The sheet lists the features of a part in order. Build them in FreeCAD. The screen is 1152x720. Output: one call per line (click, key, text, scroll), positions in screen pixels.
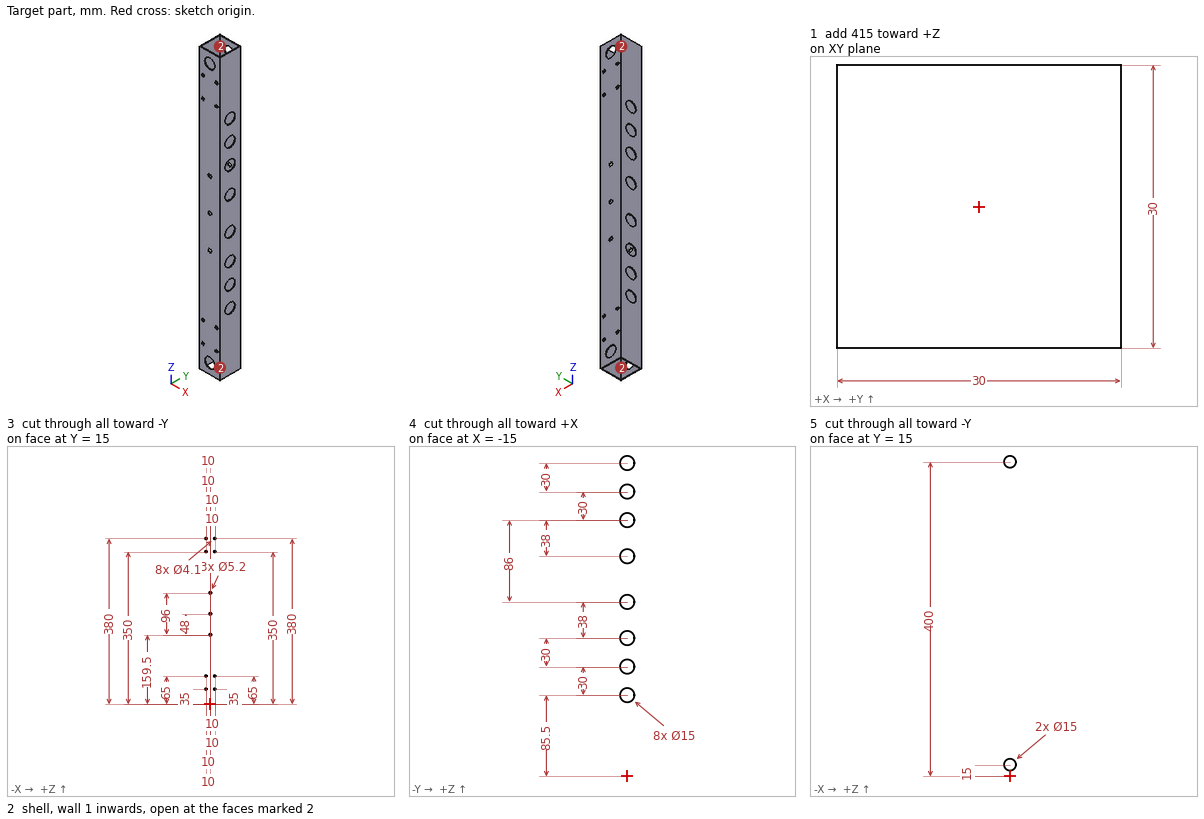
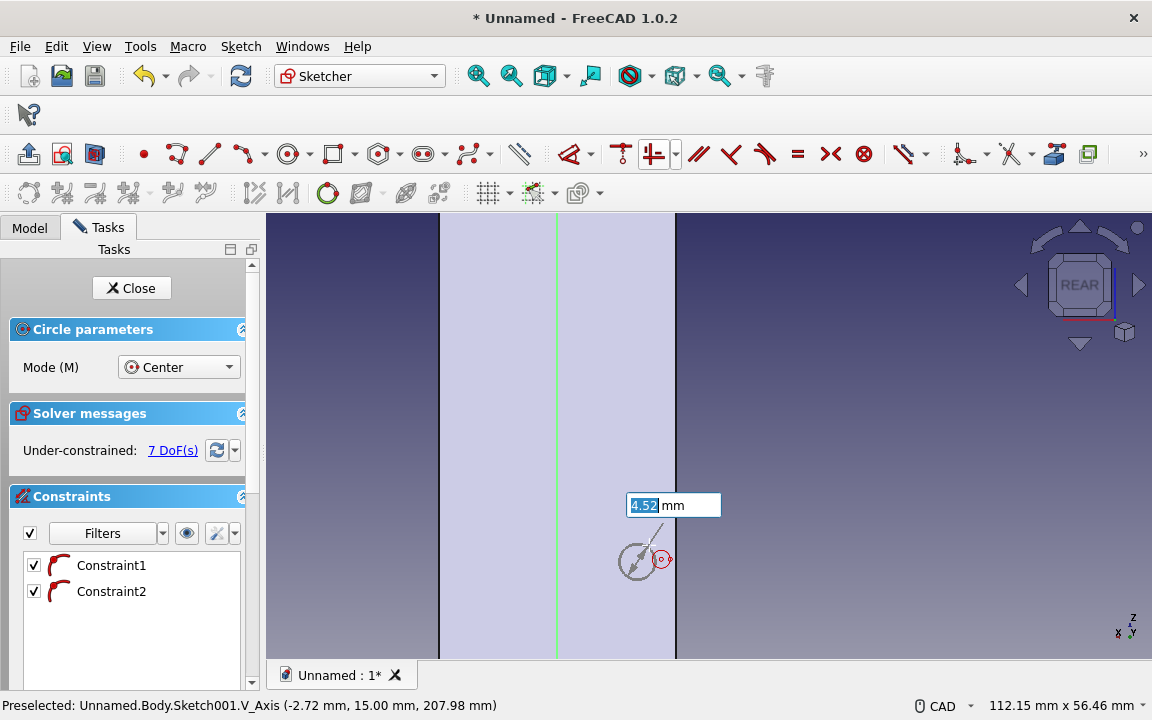
click(648, 544)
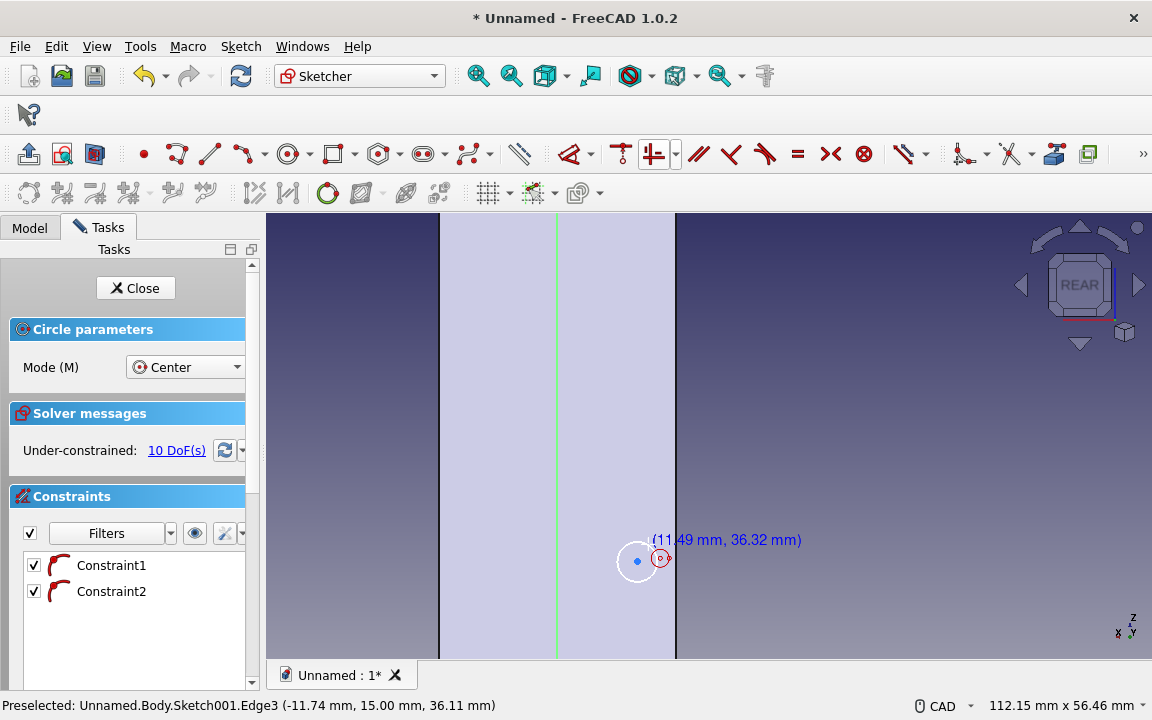
scroll(649, 547, down, 12)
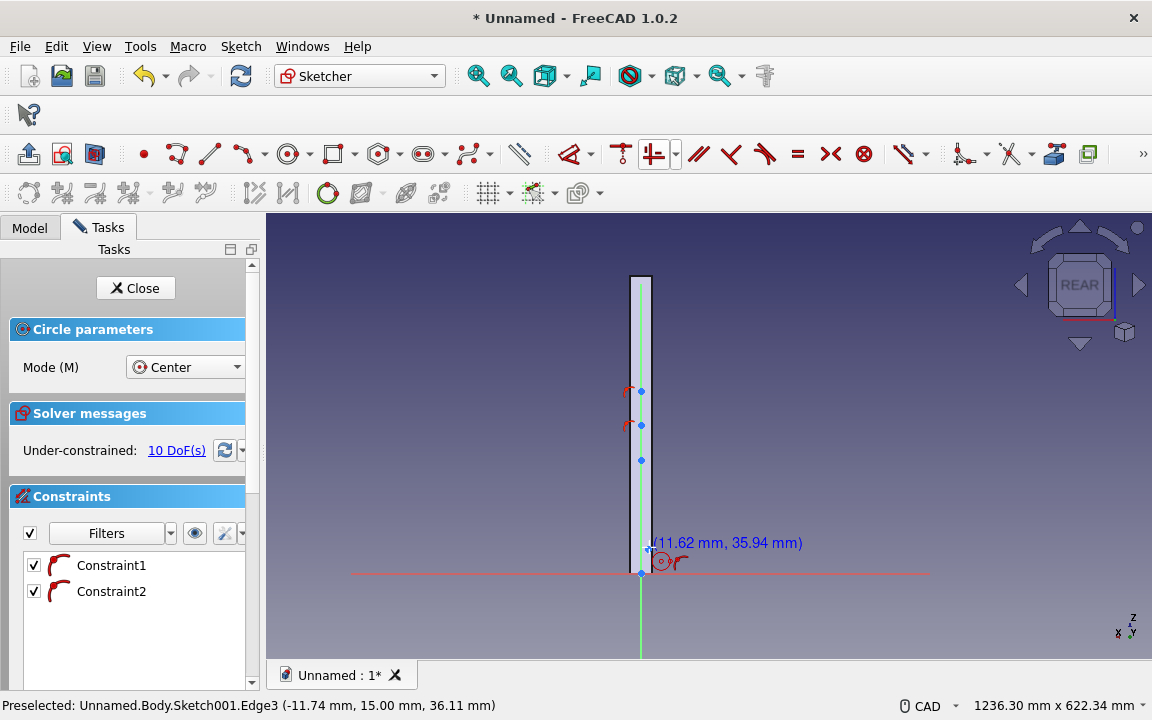
scroll(648, 301, up, 14)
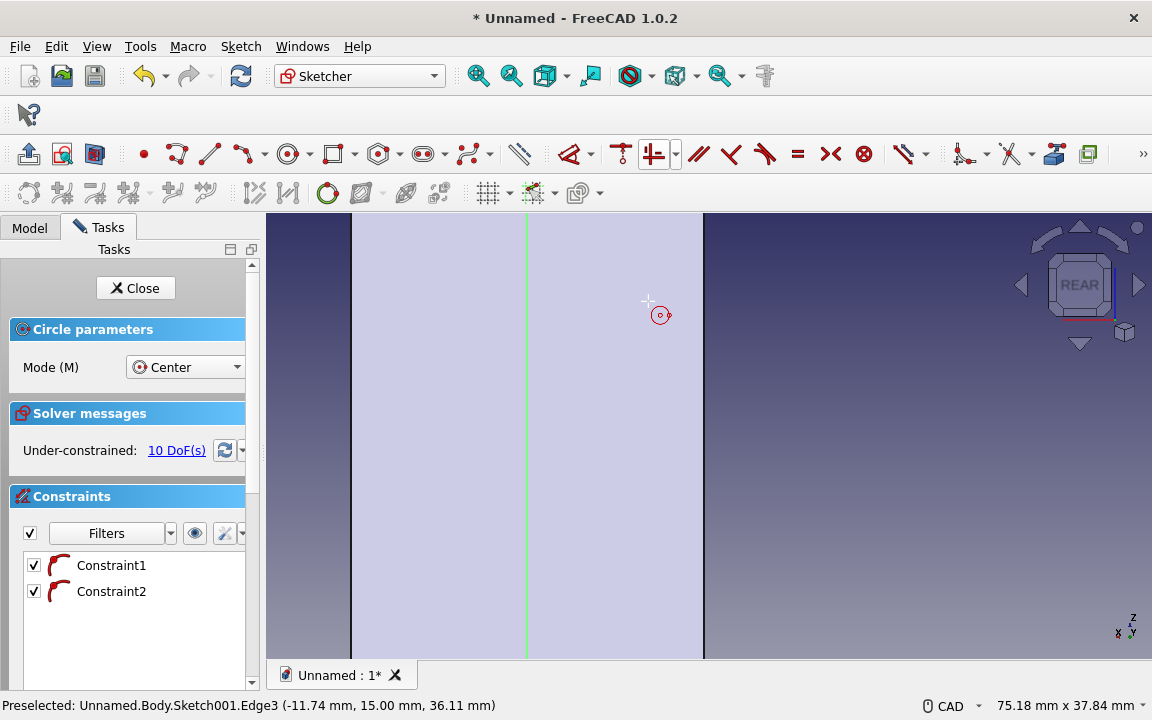
scroll(648, 301, down, 14)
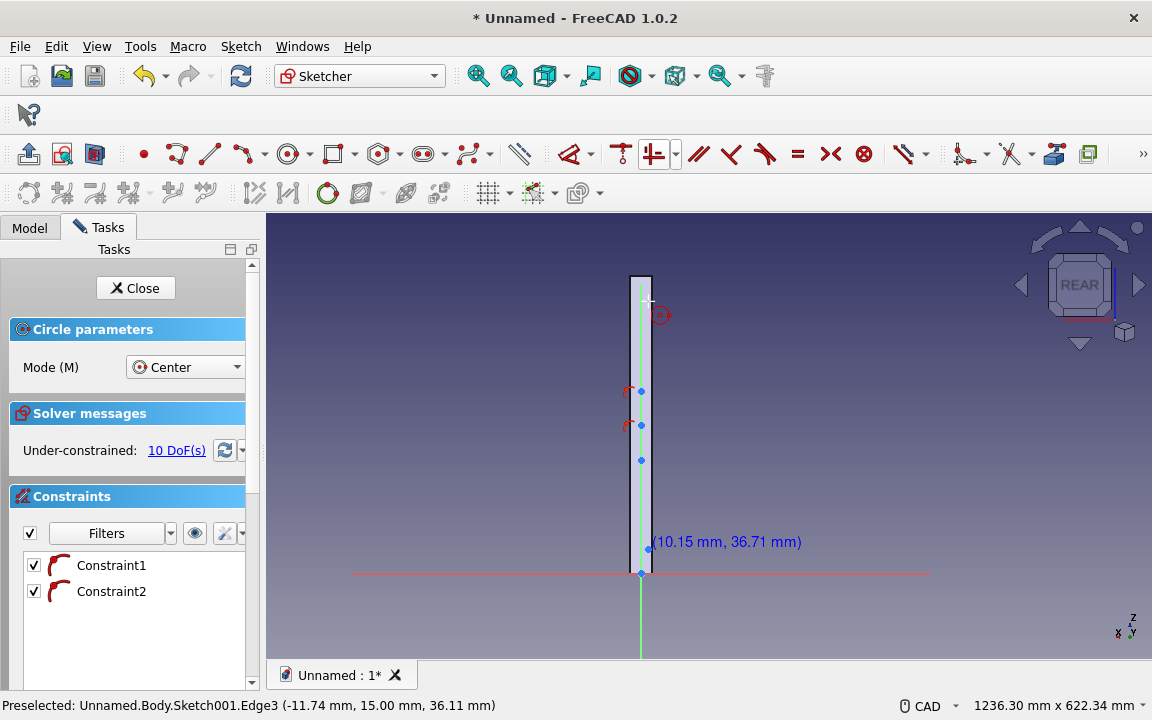
scroll(648, 301, up, 4)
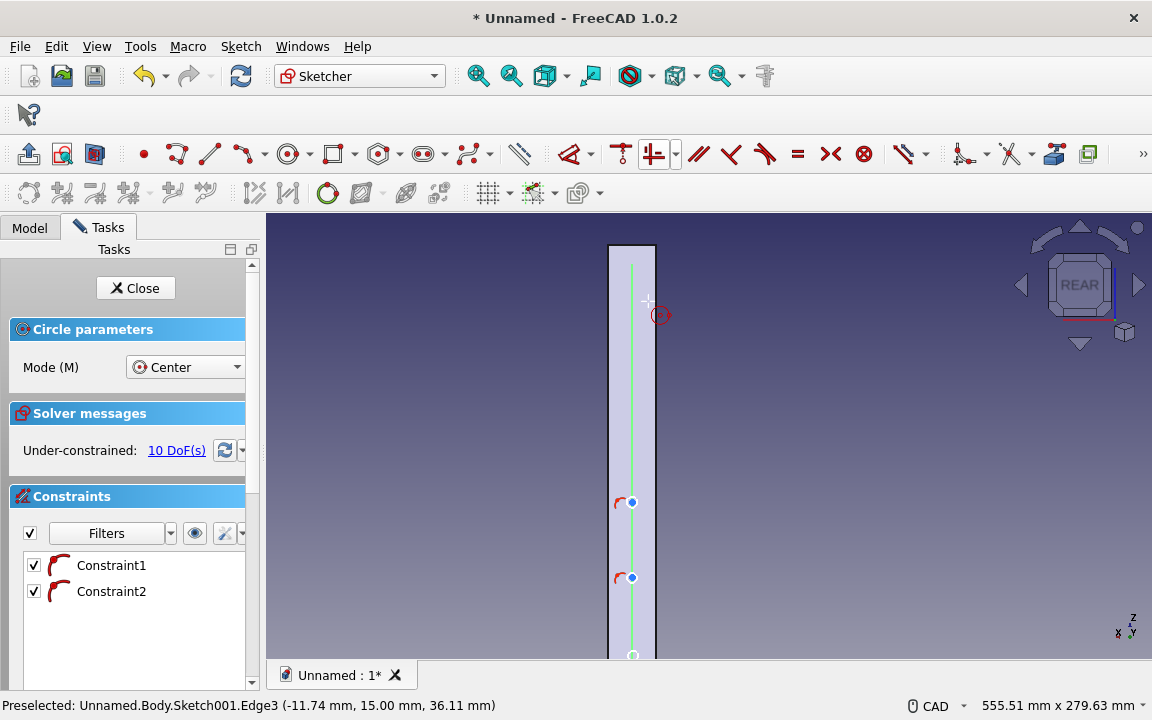
click(648, 301)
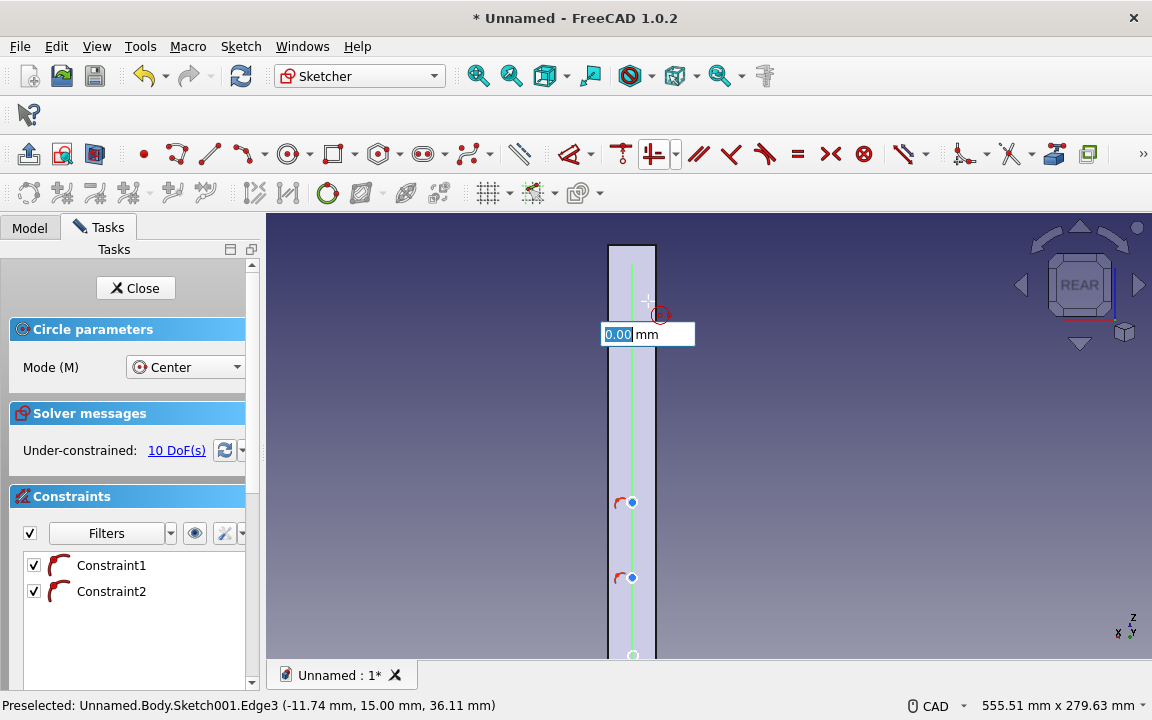
scroll(650, 299, up, 8)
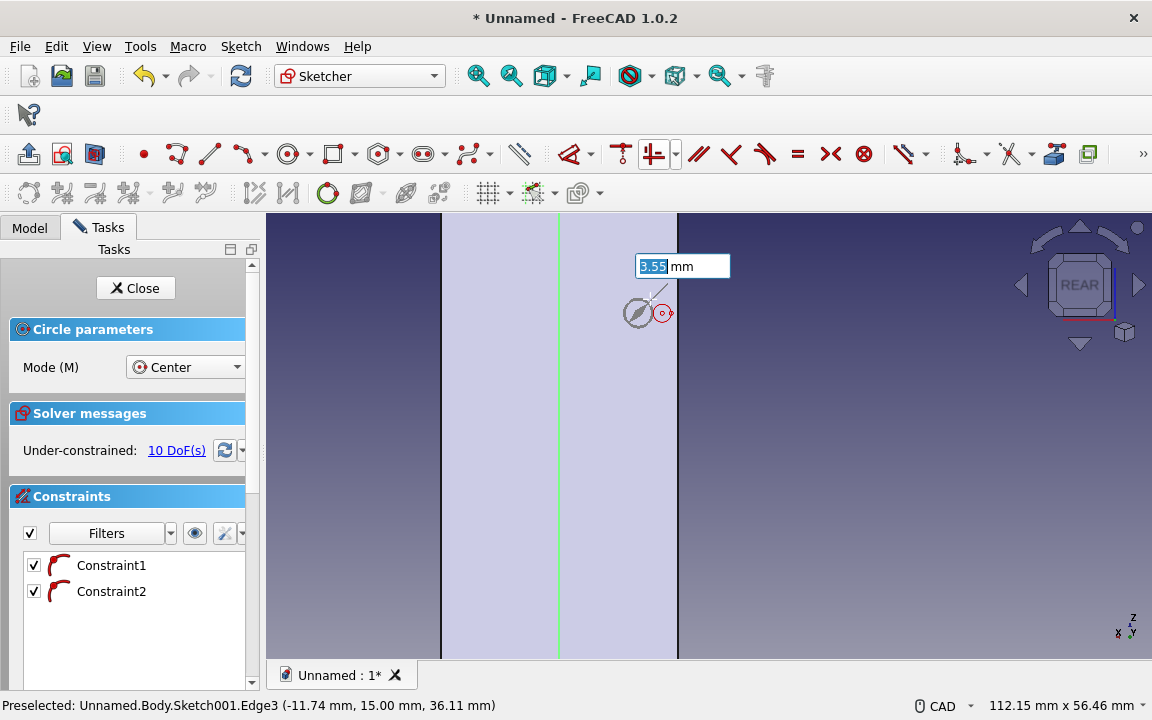
click(650, 298)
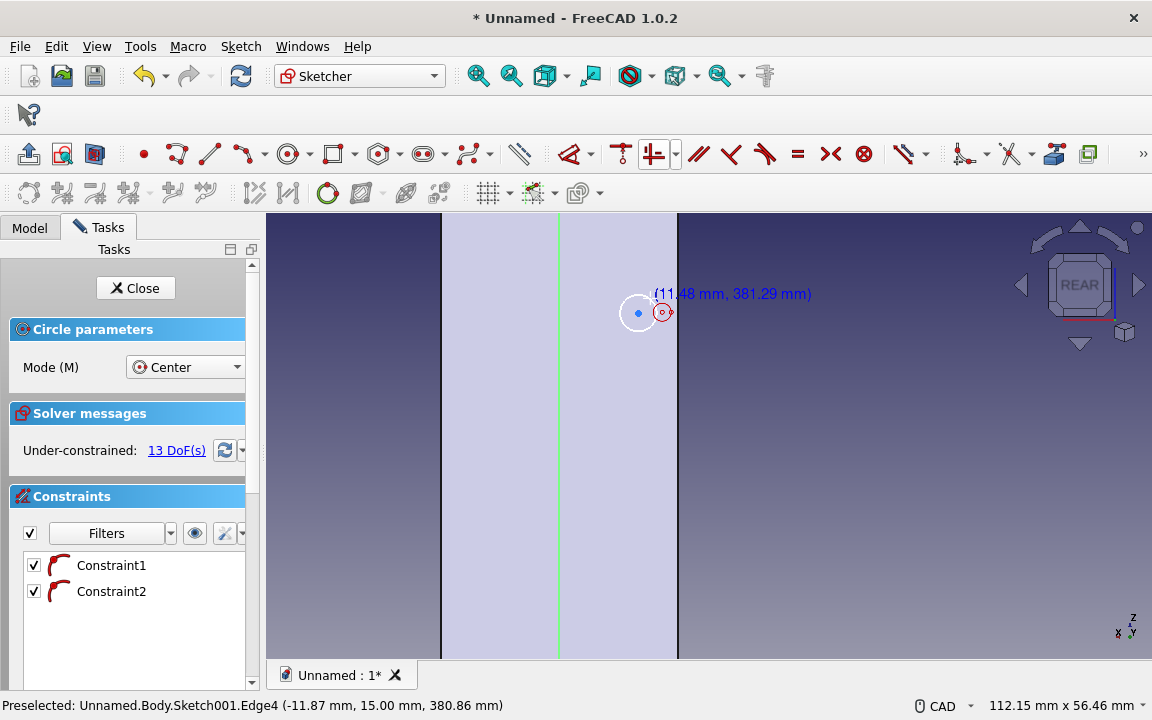
scroll(649, 300, down, 12)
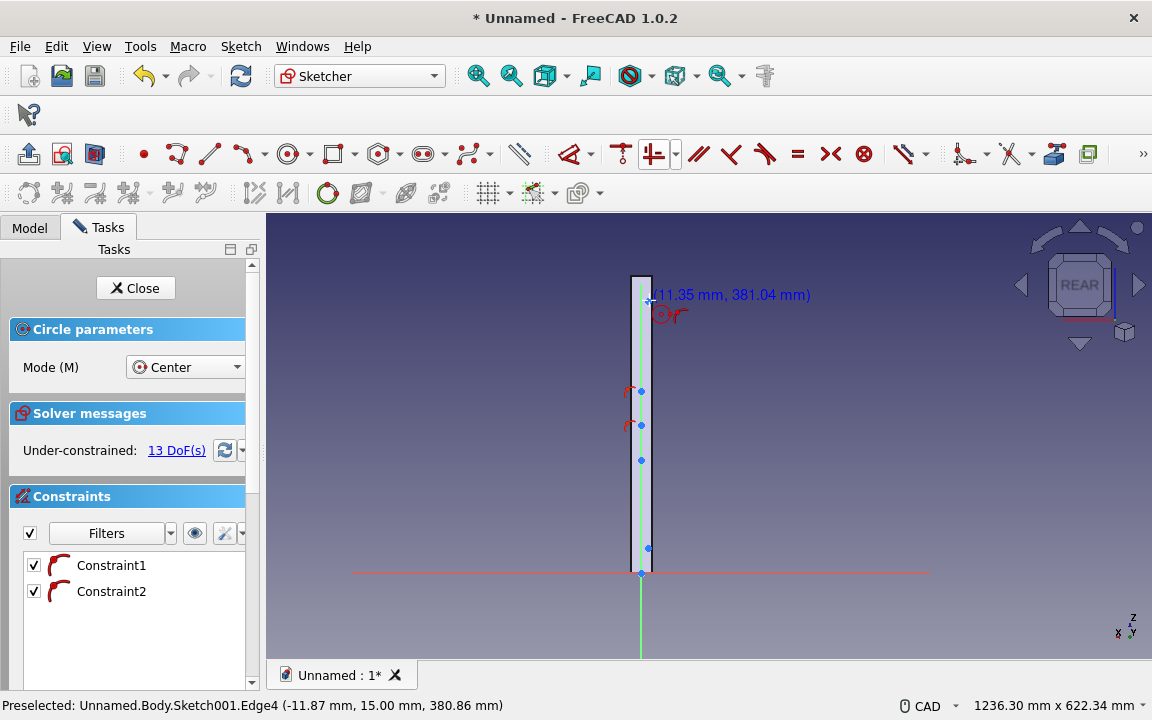
scroll(648, 527, up, 14)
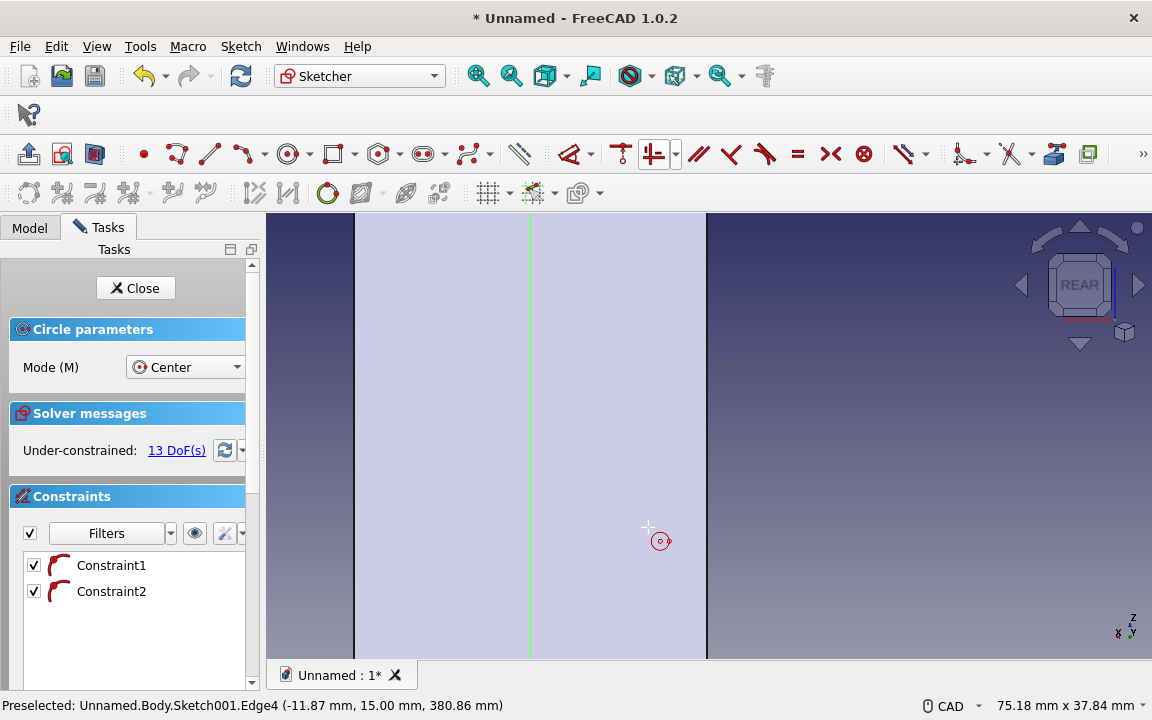
scroll(648, 527, down, 14)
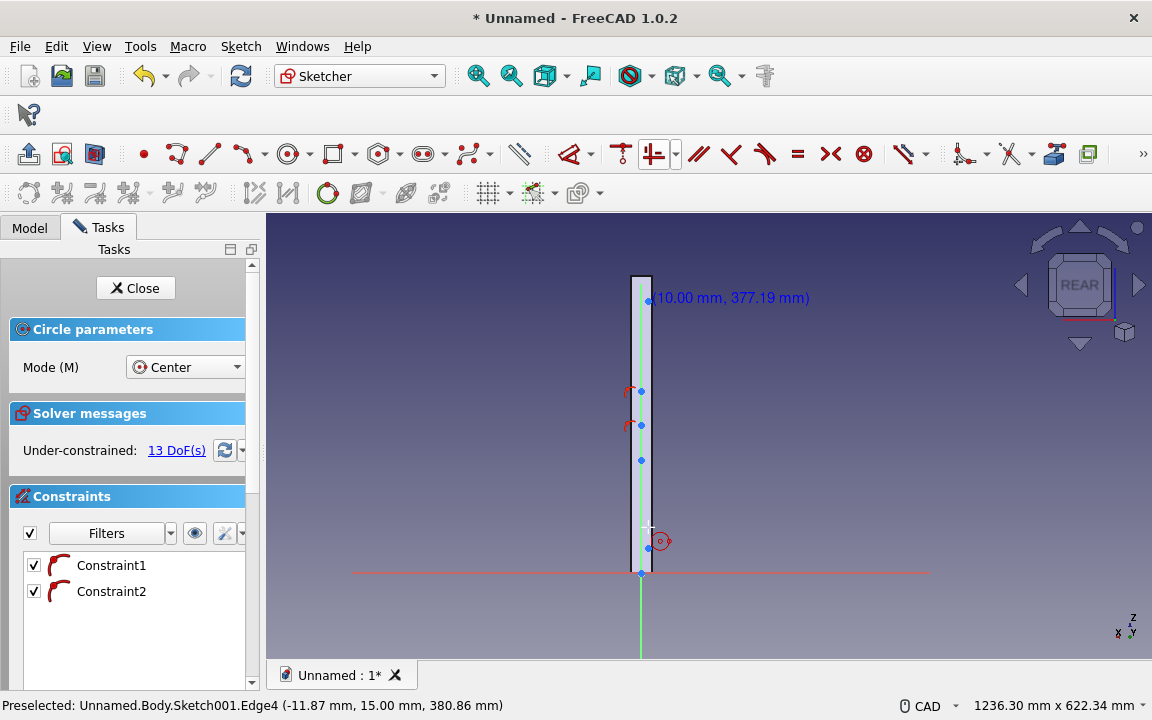
scroll(648, 527, up, 4)